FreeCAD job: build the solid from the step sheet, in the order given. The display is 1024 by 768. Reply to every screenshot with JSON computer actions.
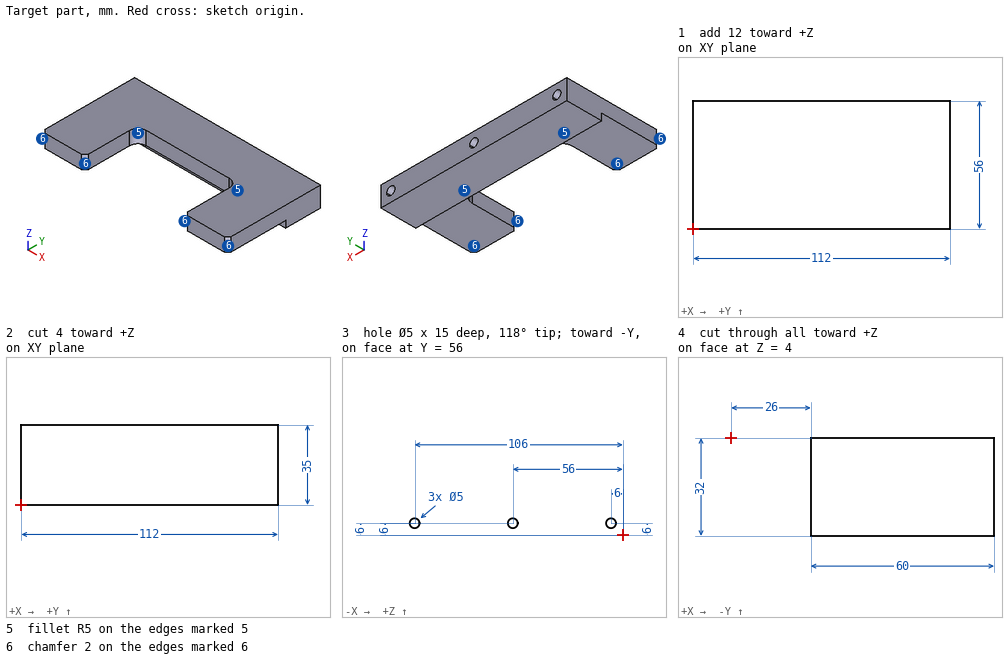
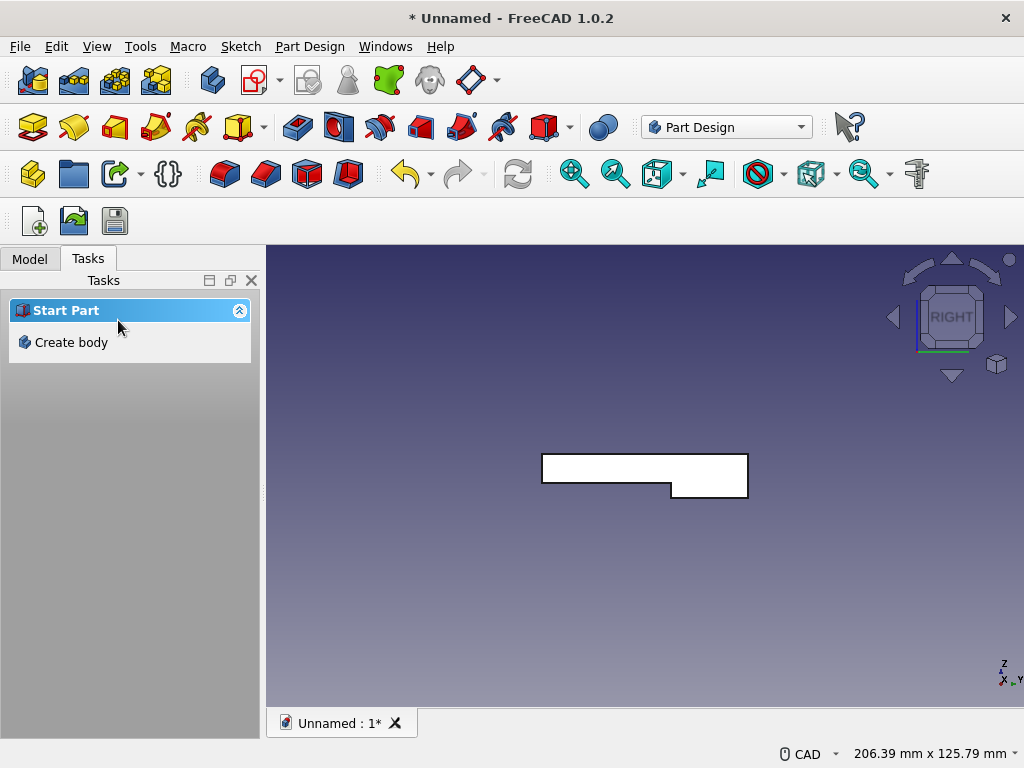
{"action": "left_click", "coordinate": [575, 174]}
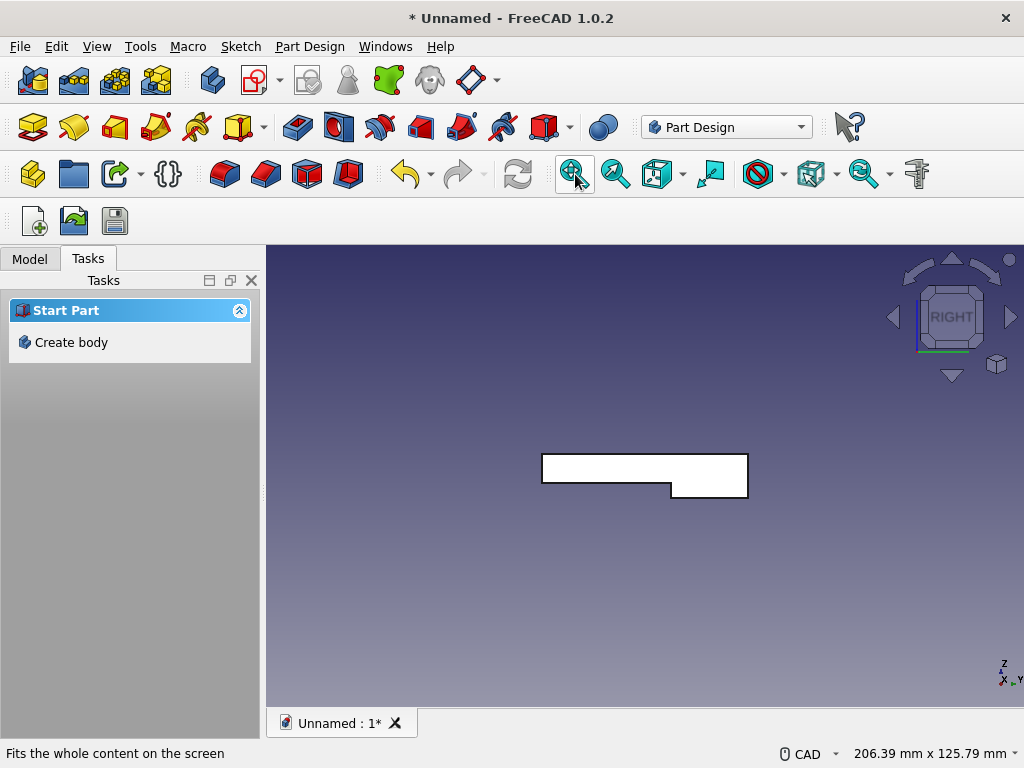
{"action": "key", "text": "5"}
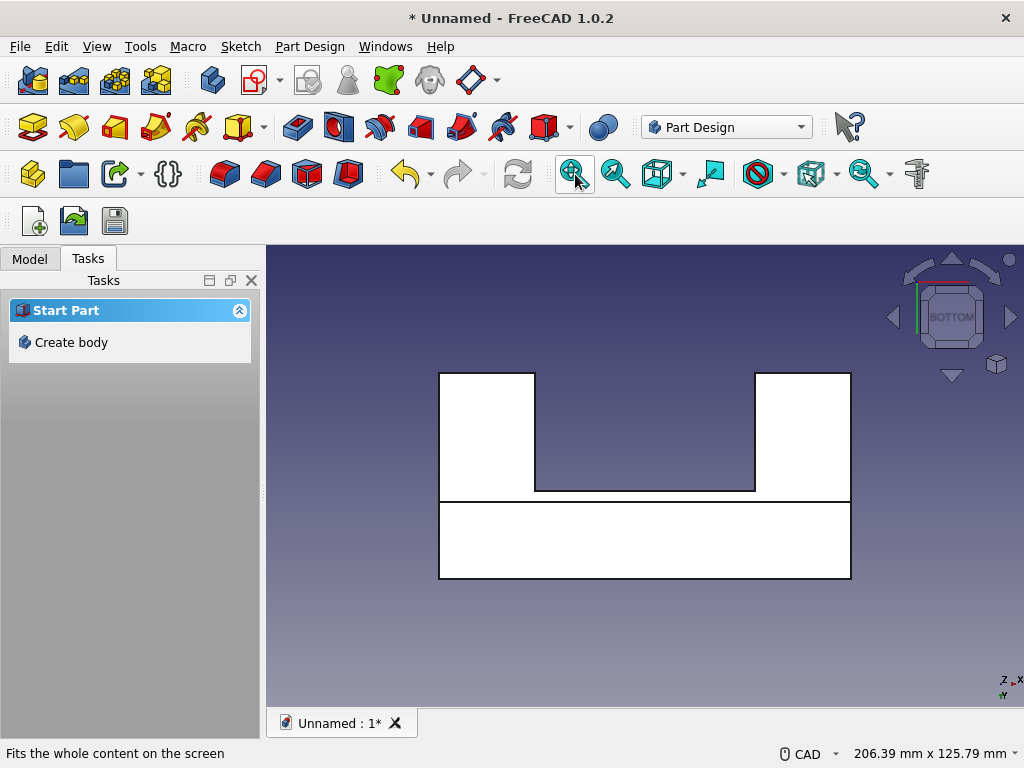
{"action": "key", "text": "4"}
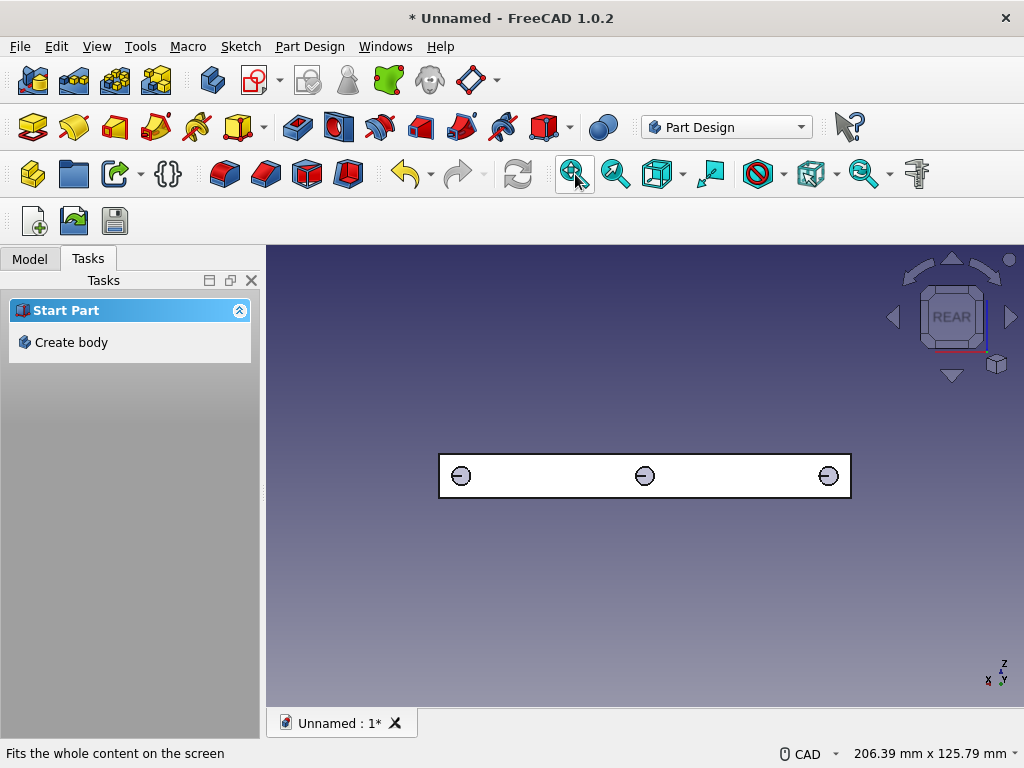
{"action": "key", "text": "6"}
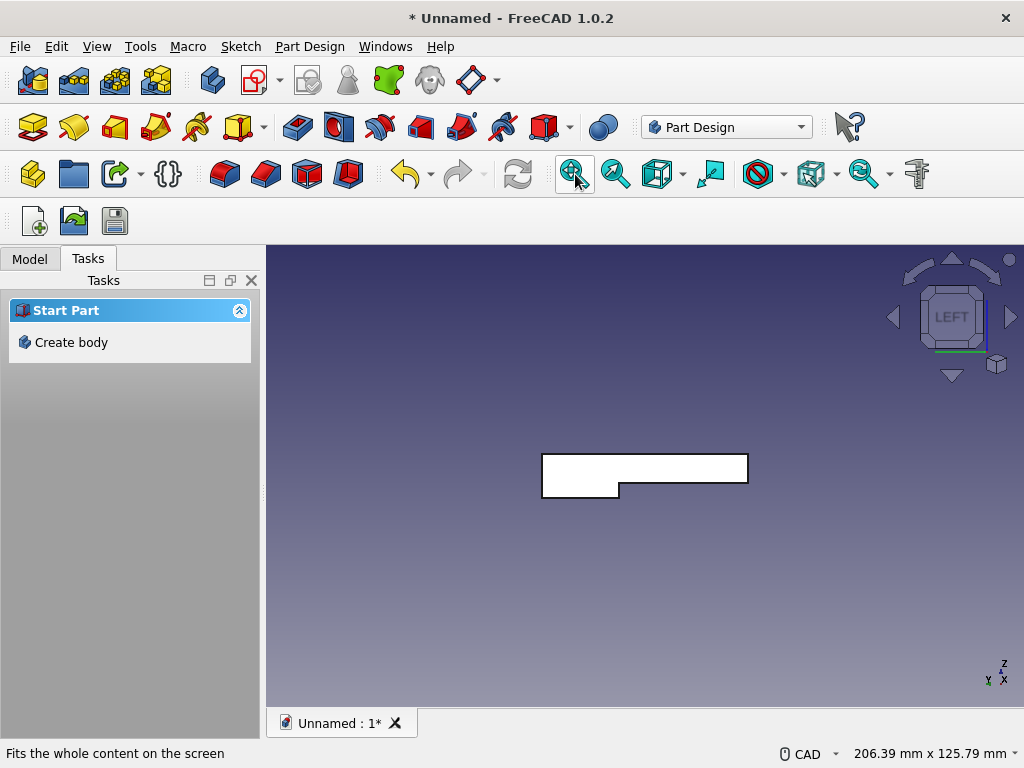
{"action": "left_click", "coordinate": [575, 174]}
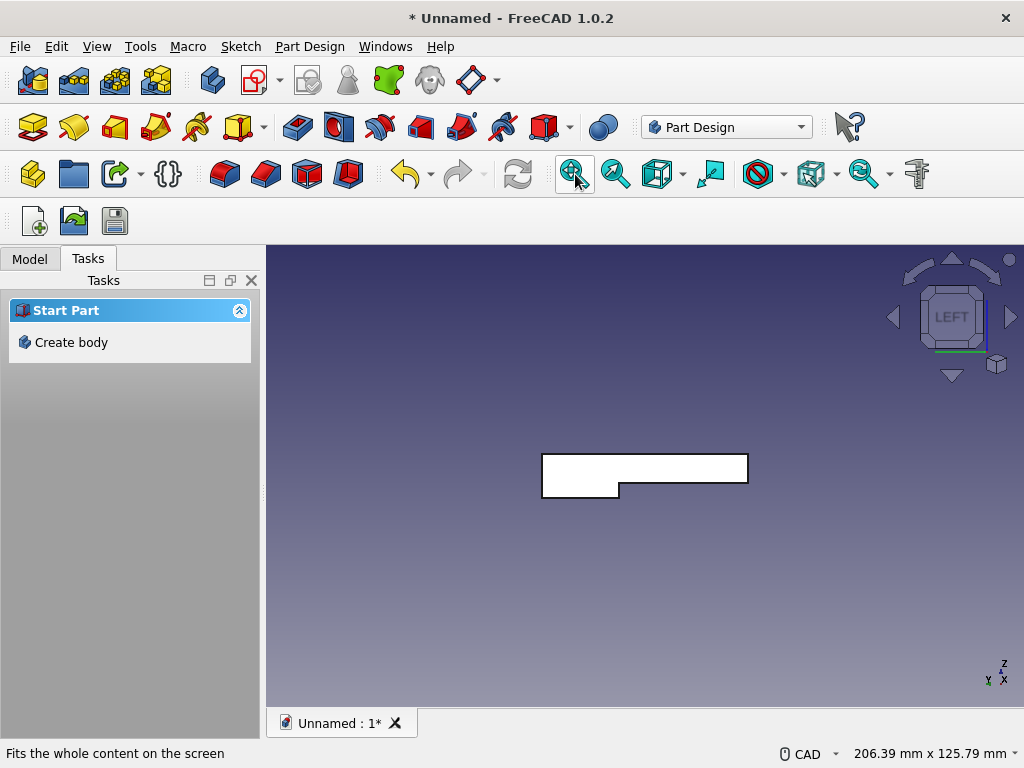
{"action": "key", "text": "v 3"}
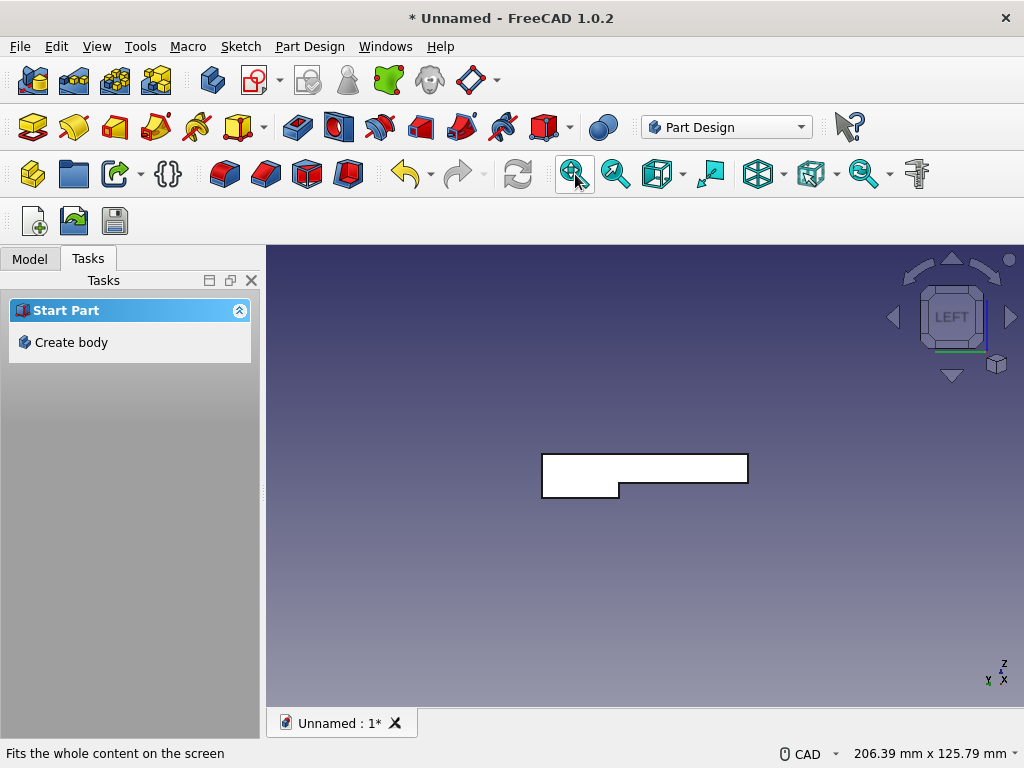
{"action": "key", "text": "0"}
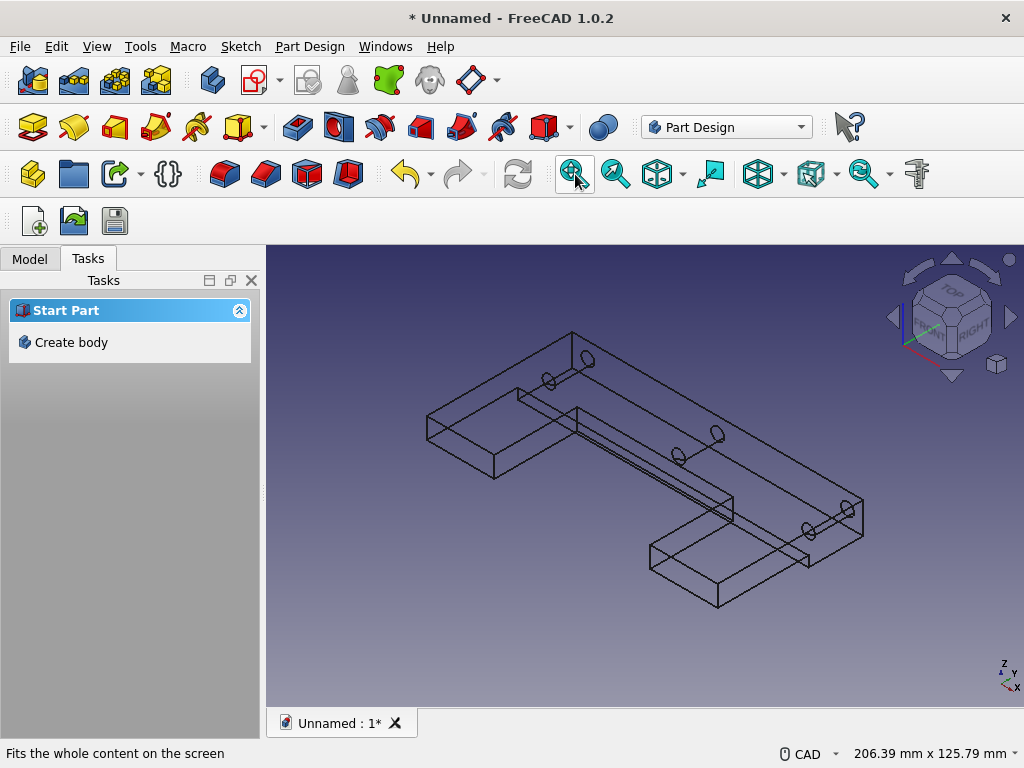
{"action": "left_click", "coordinate": [733, 508]}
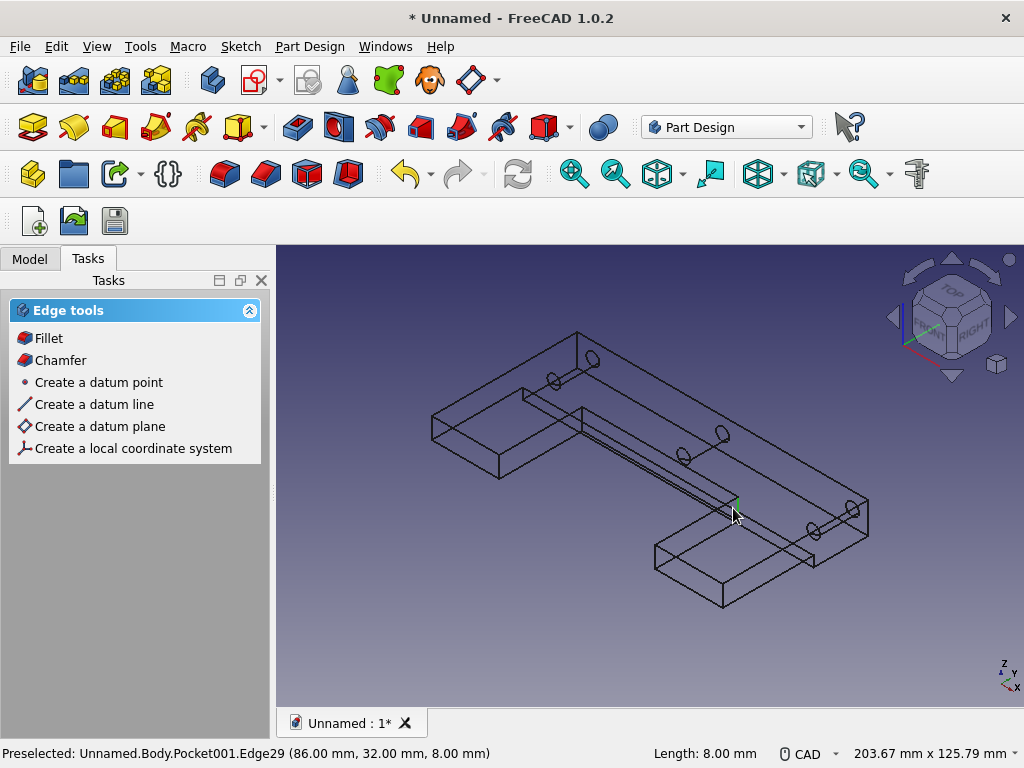
{"action": "left_click", "coordinate": [582, 418], "text": "ctrl"}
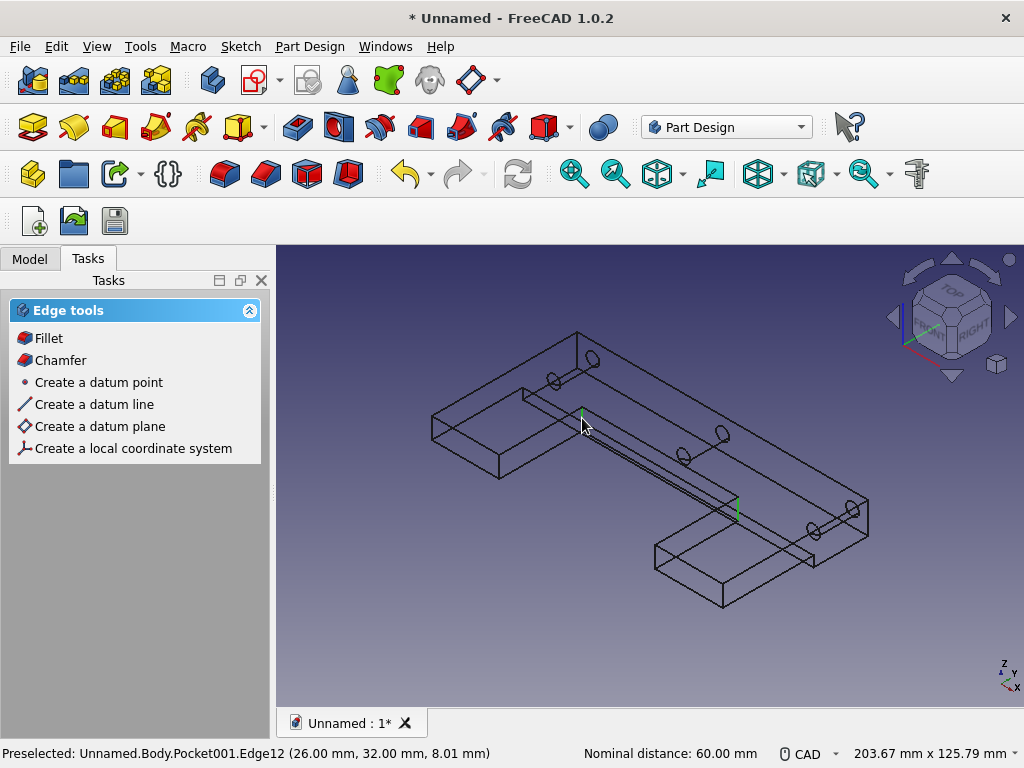
{"action": "key", "text": "v 1"}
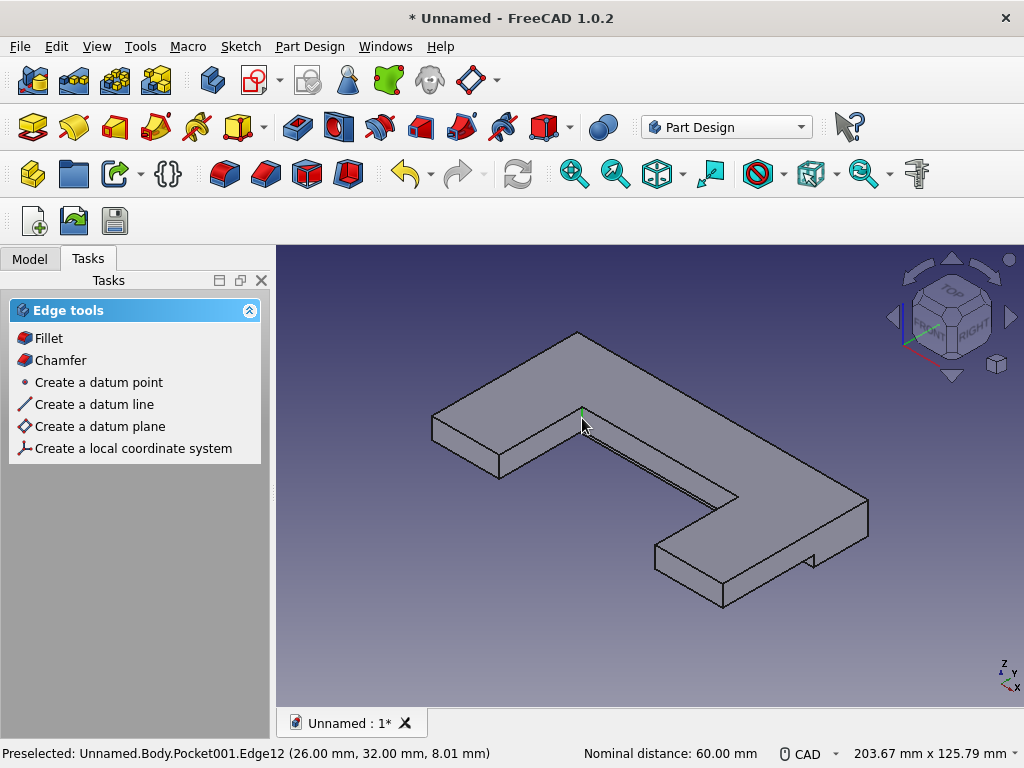
{"action": "left_click", "coordinate": [225, 174]}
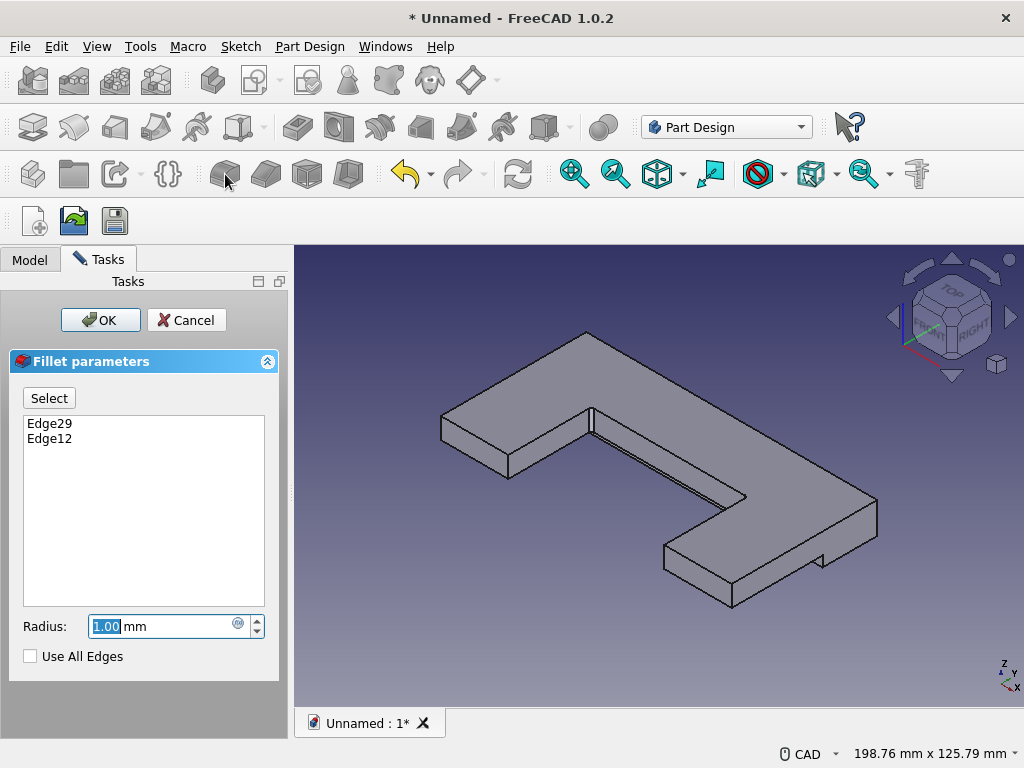
{"action": "type", "text": "5"}
{"action": "key", "text": "Tab"}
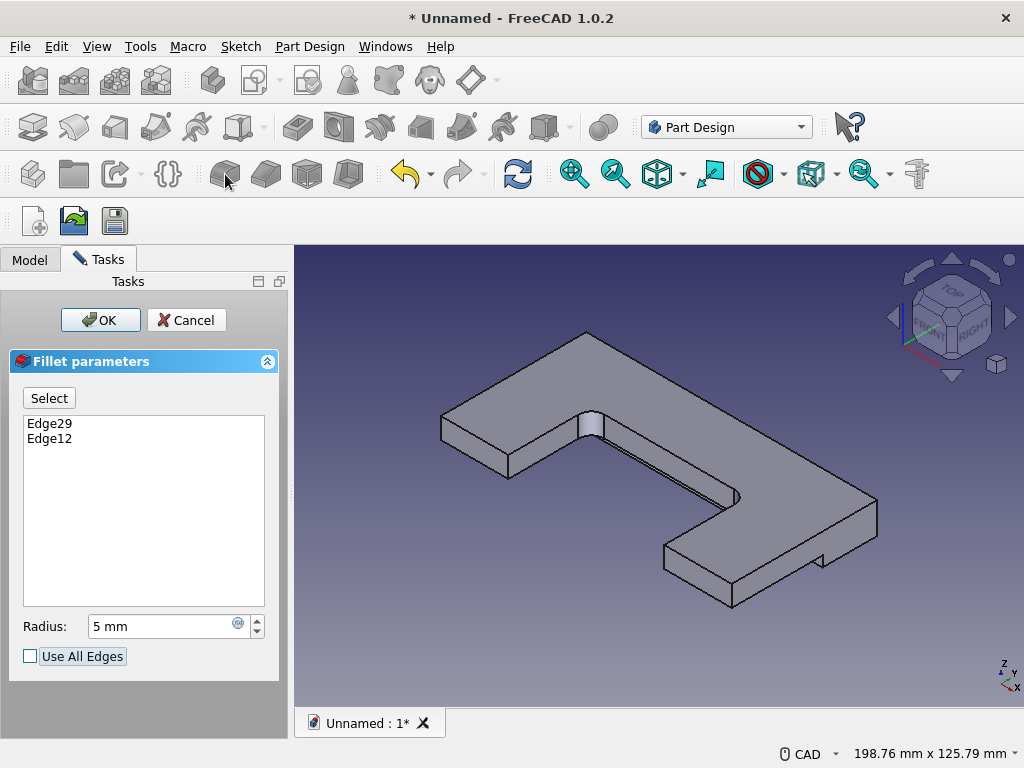
{"action": "left_click", "coordinate": [101, 320]}